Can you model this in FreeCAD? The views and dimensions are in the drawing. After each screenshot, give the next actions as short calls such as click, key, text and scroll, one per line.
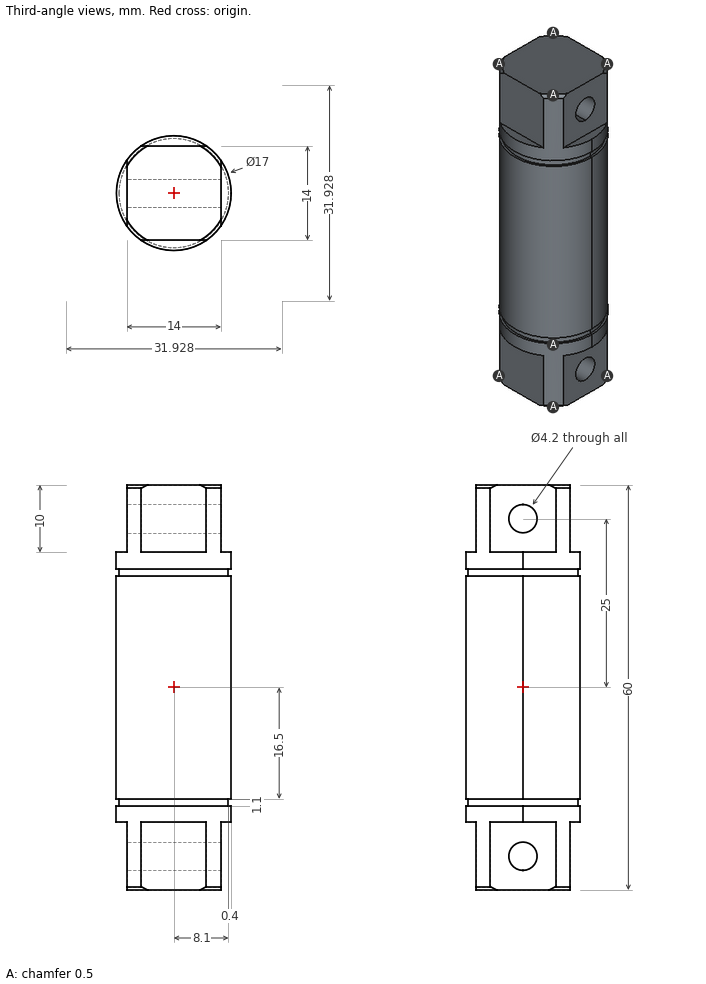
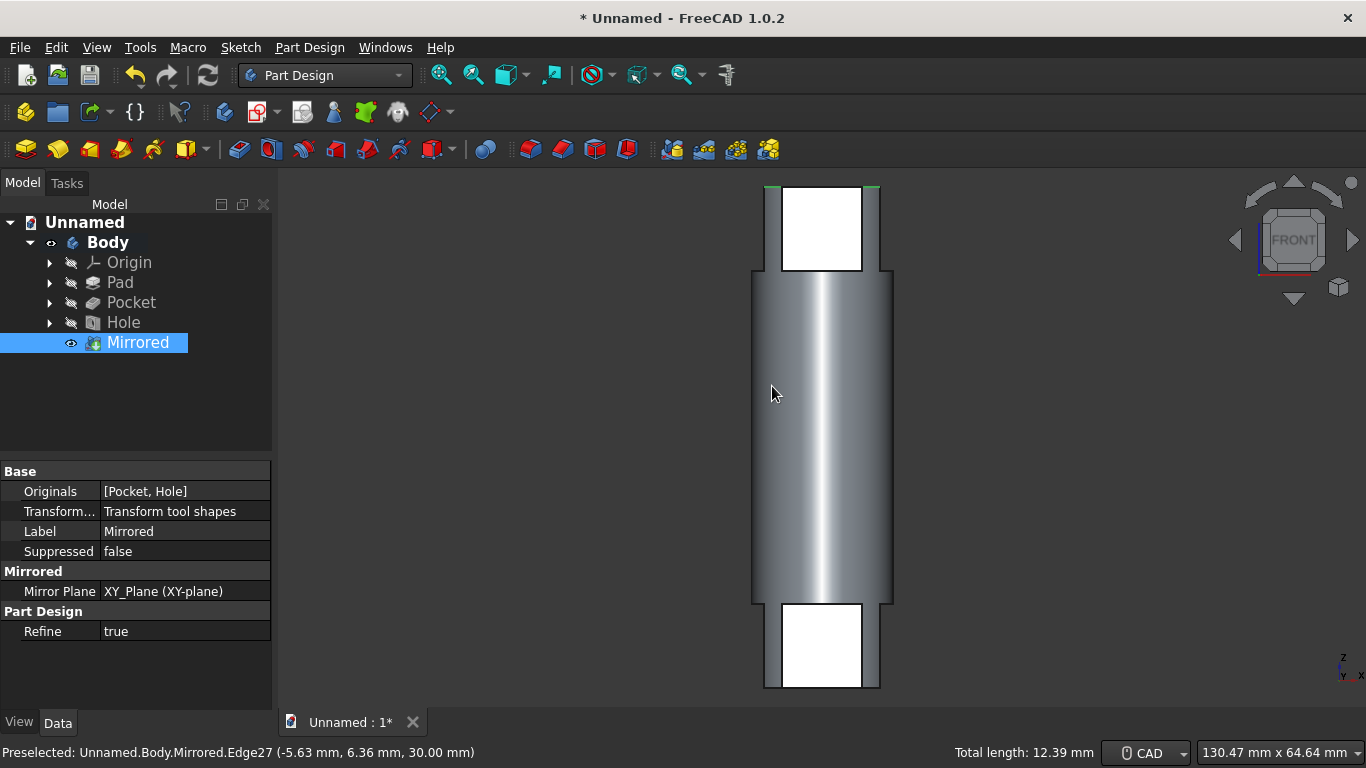
key(3)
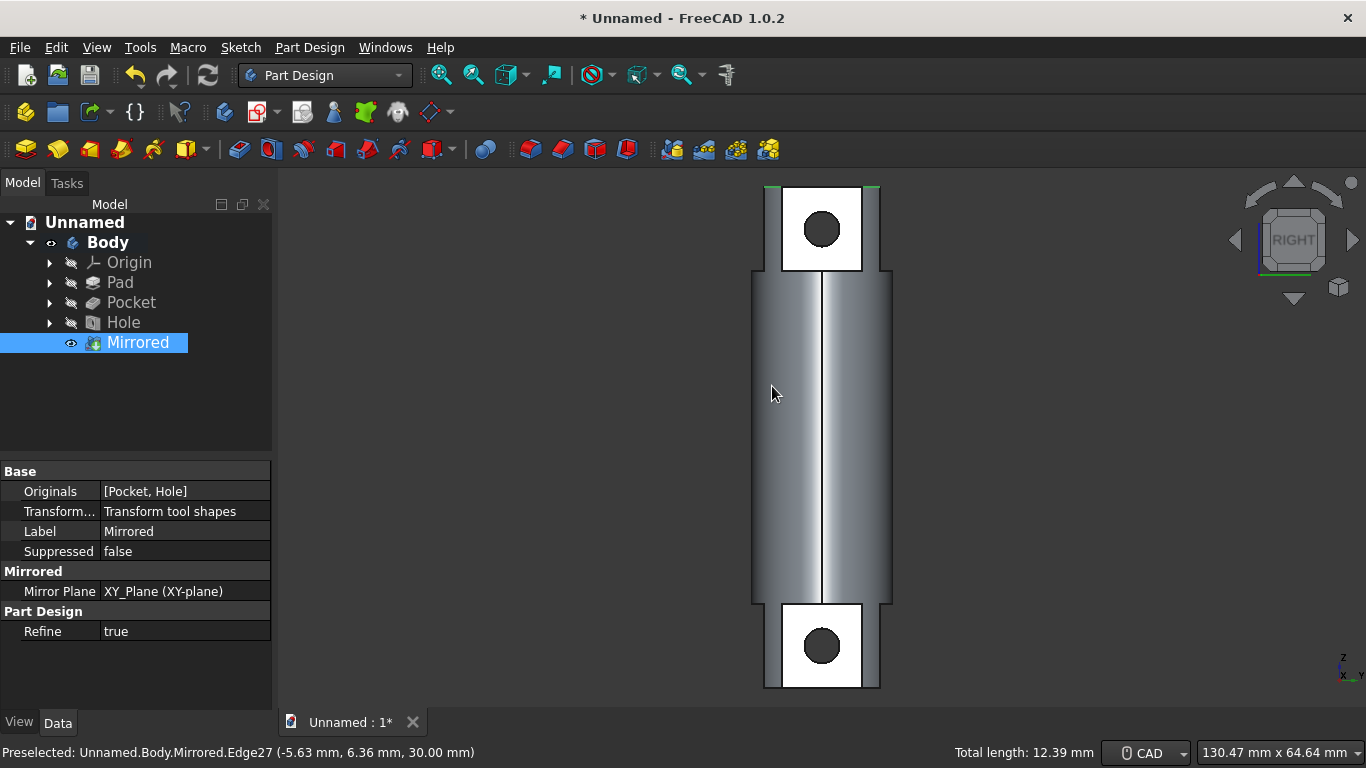
key(5)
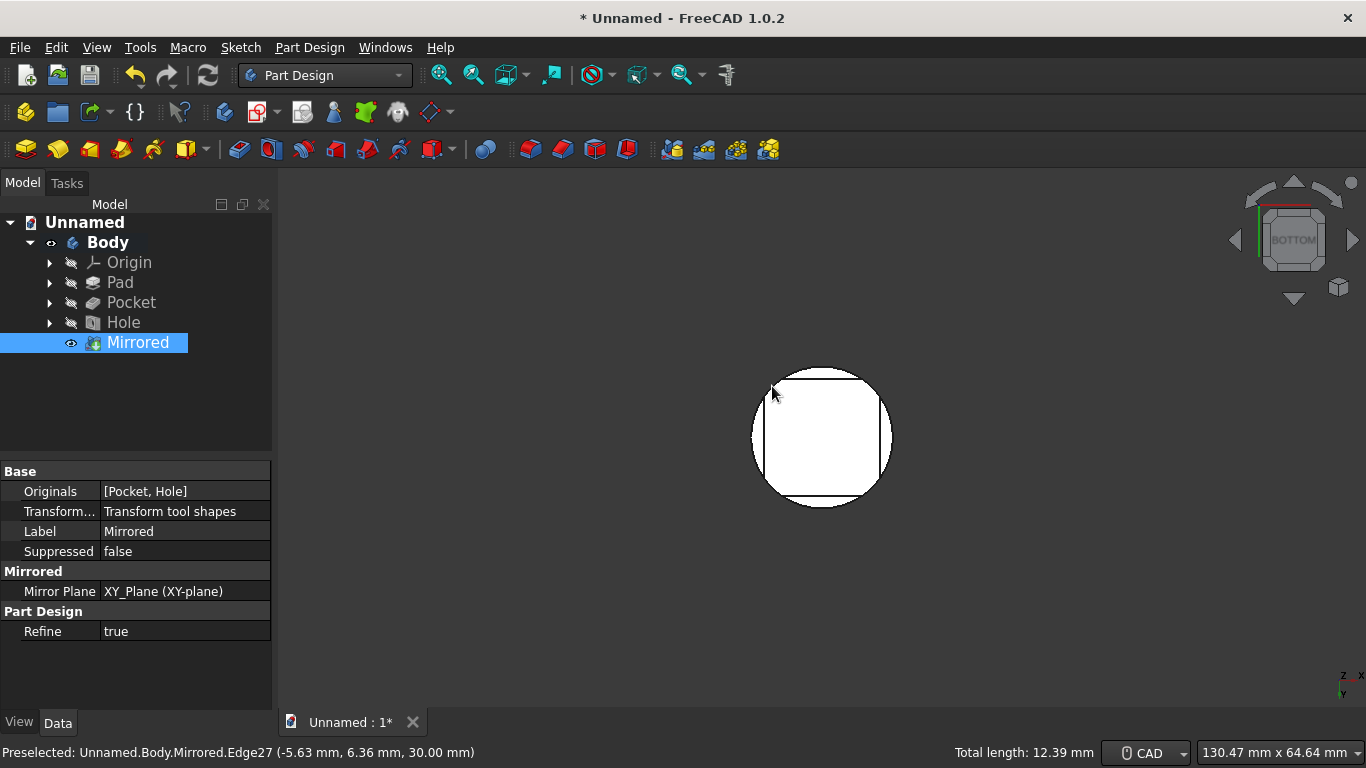
click(442, 76)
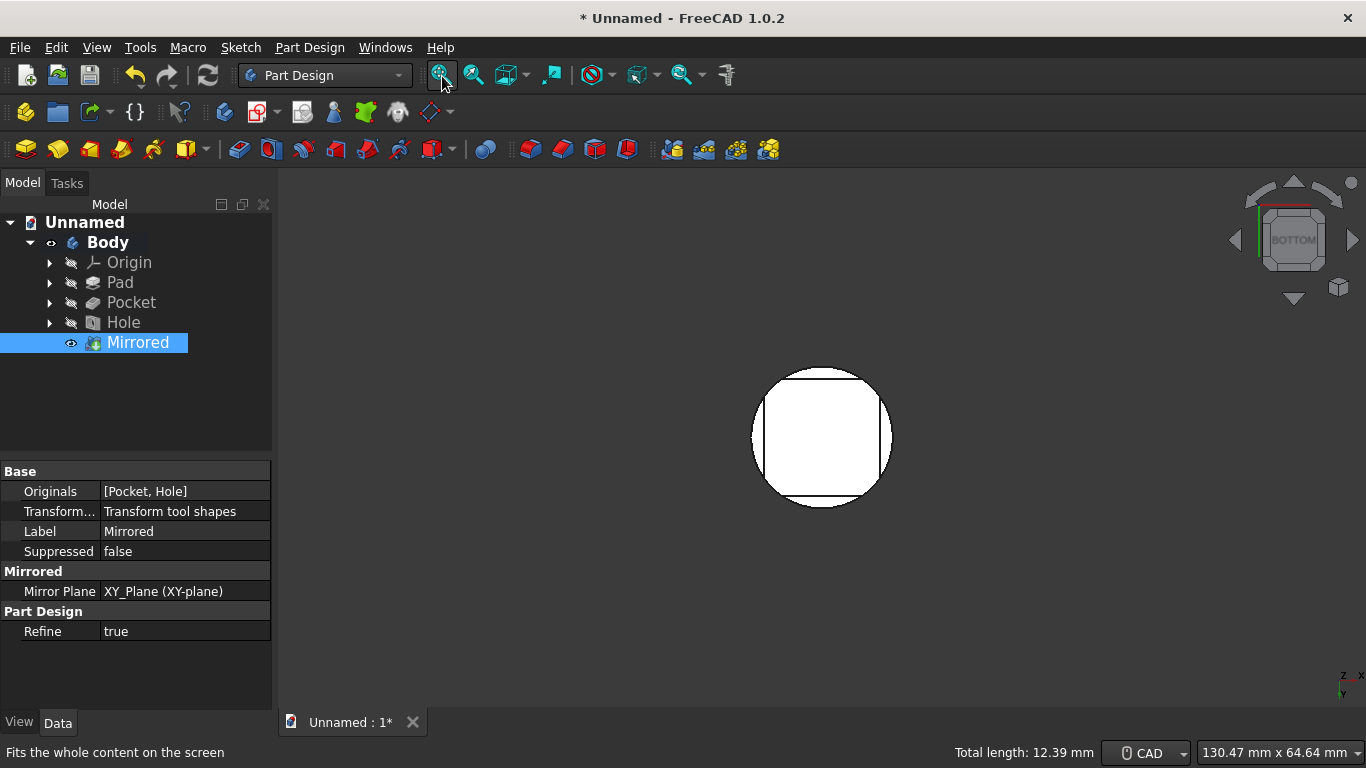
click(872, 487, ctrl)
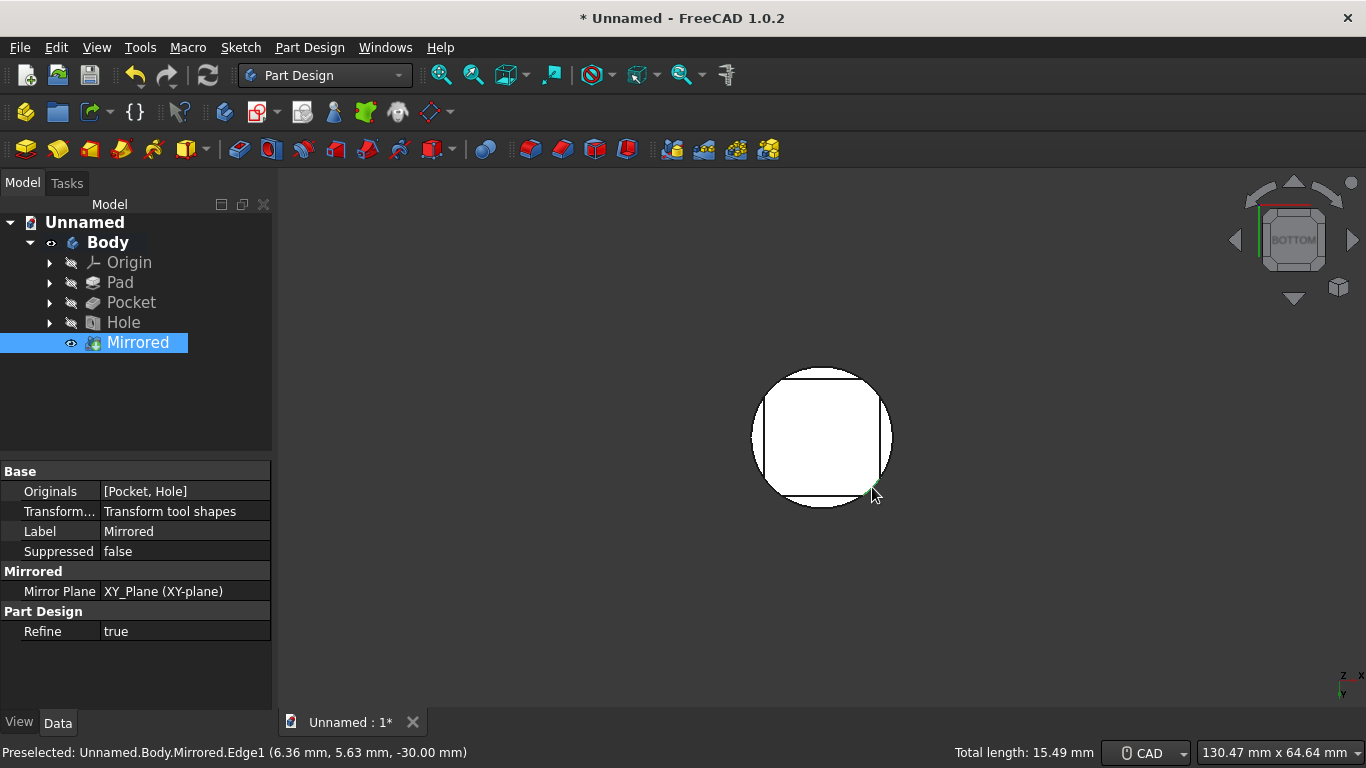
click(772, 487, ctrl)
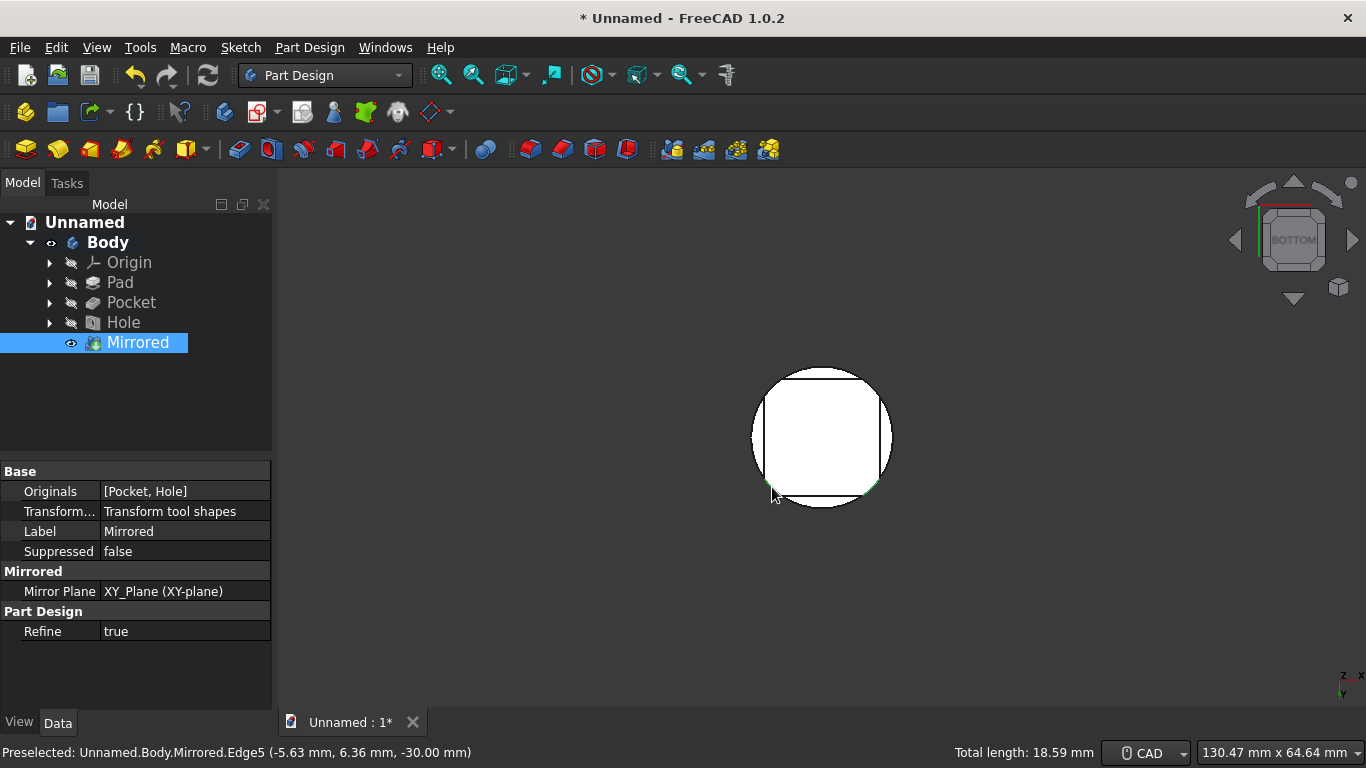
click(772, 386, ctrl)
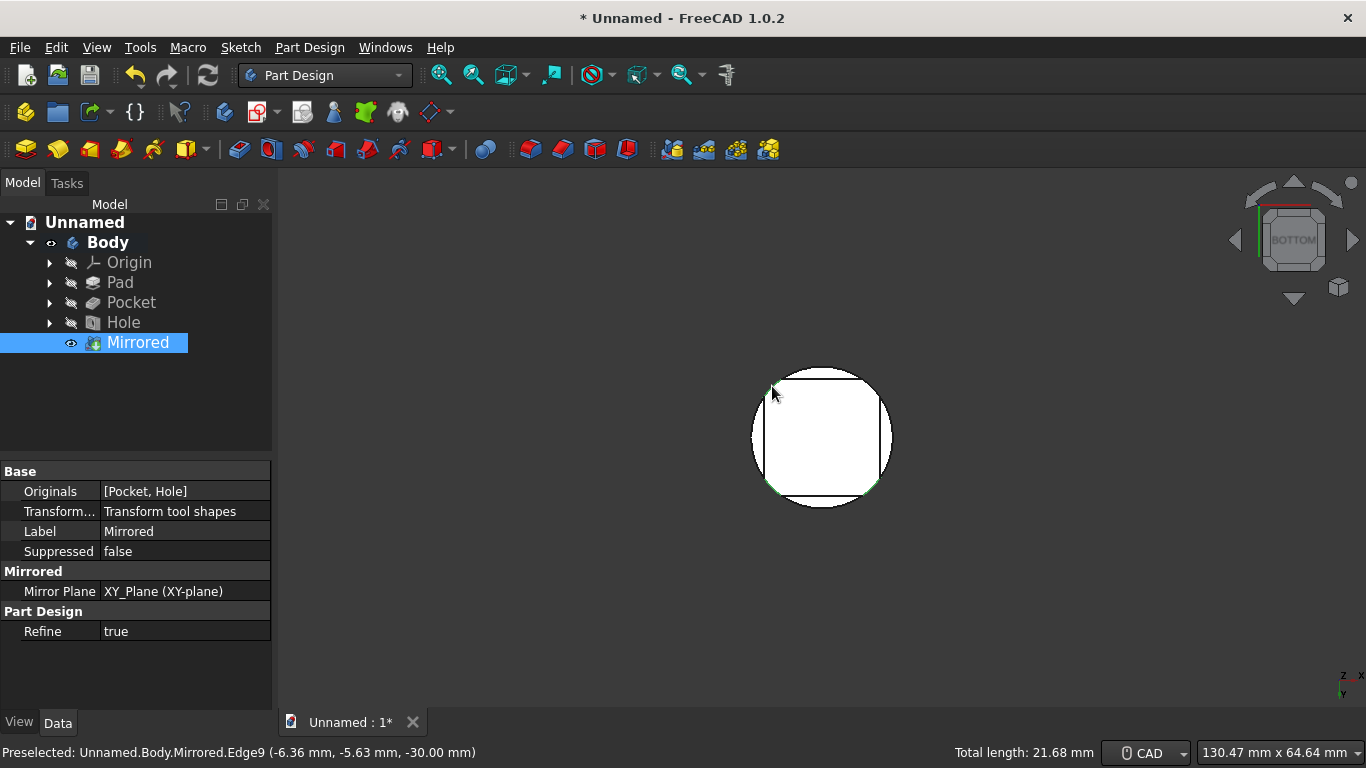
click(872, 386, ctrl)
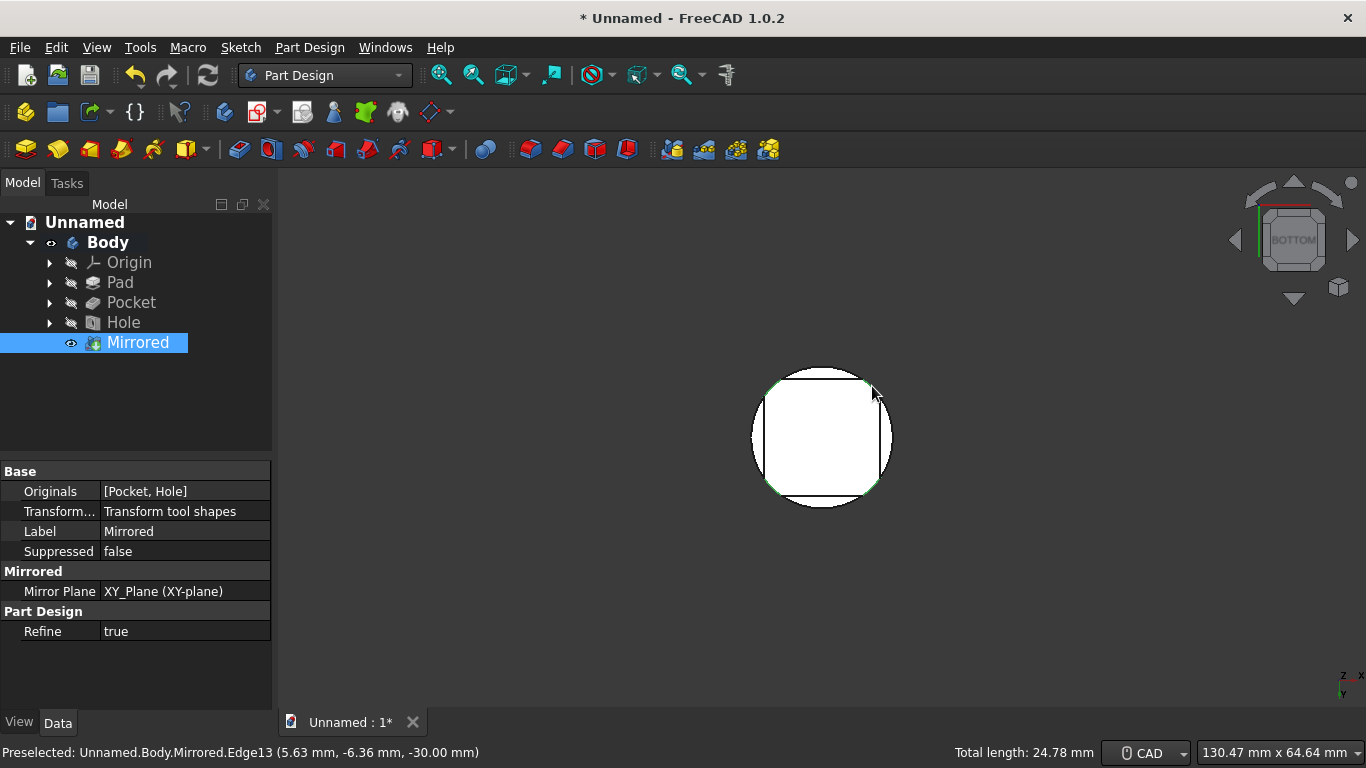
click(564, 150)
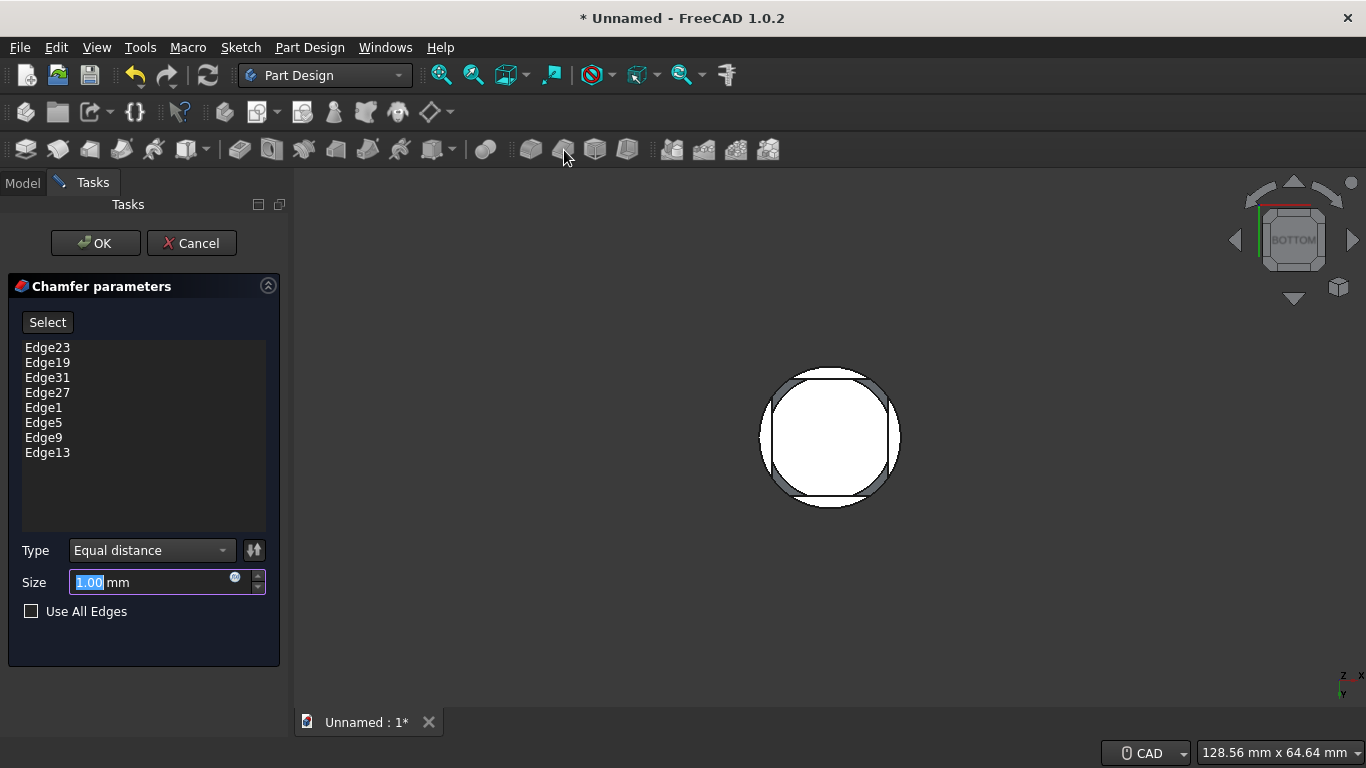
text(0.5)
key(Tab)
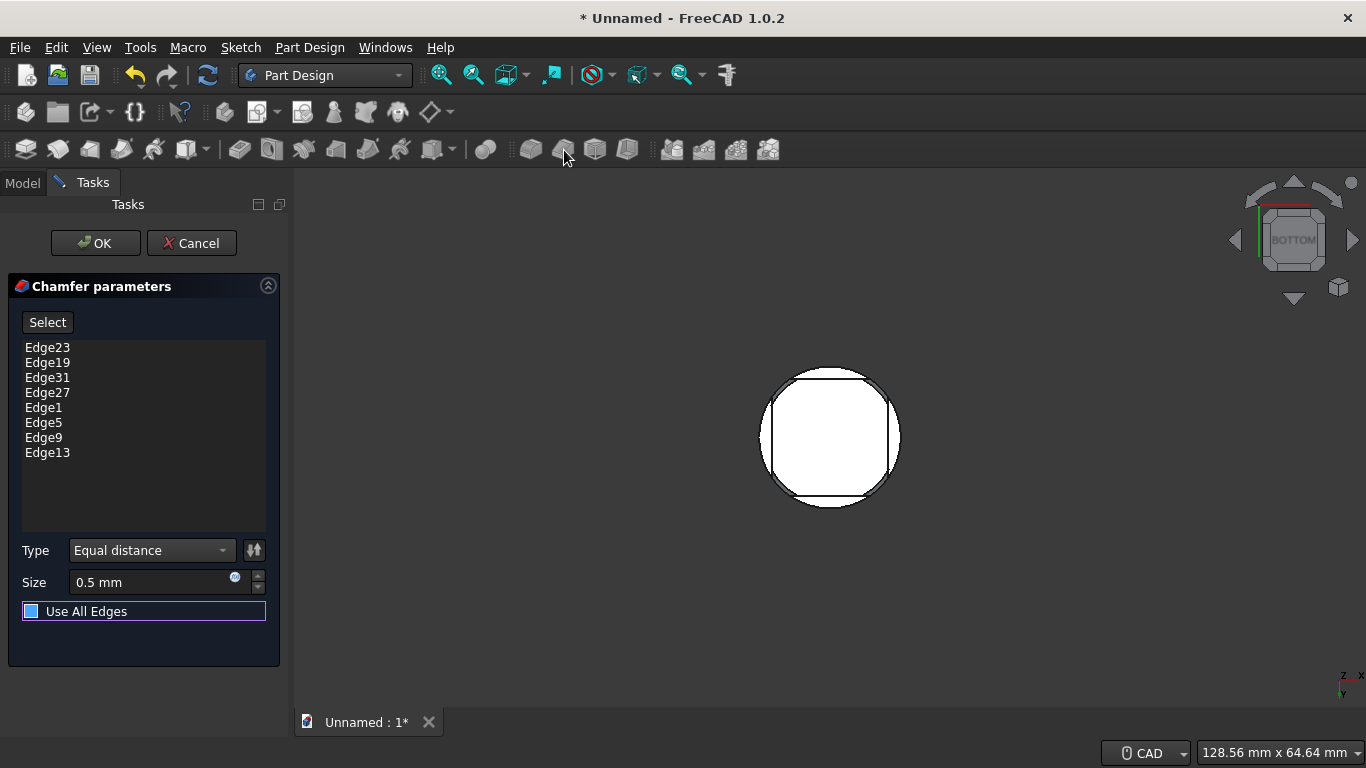
click(96, 243)